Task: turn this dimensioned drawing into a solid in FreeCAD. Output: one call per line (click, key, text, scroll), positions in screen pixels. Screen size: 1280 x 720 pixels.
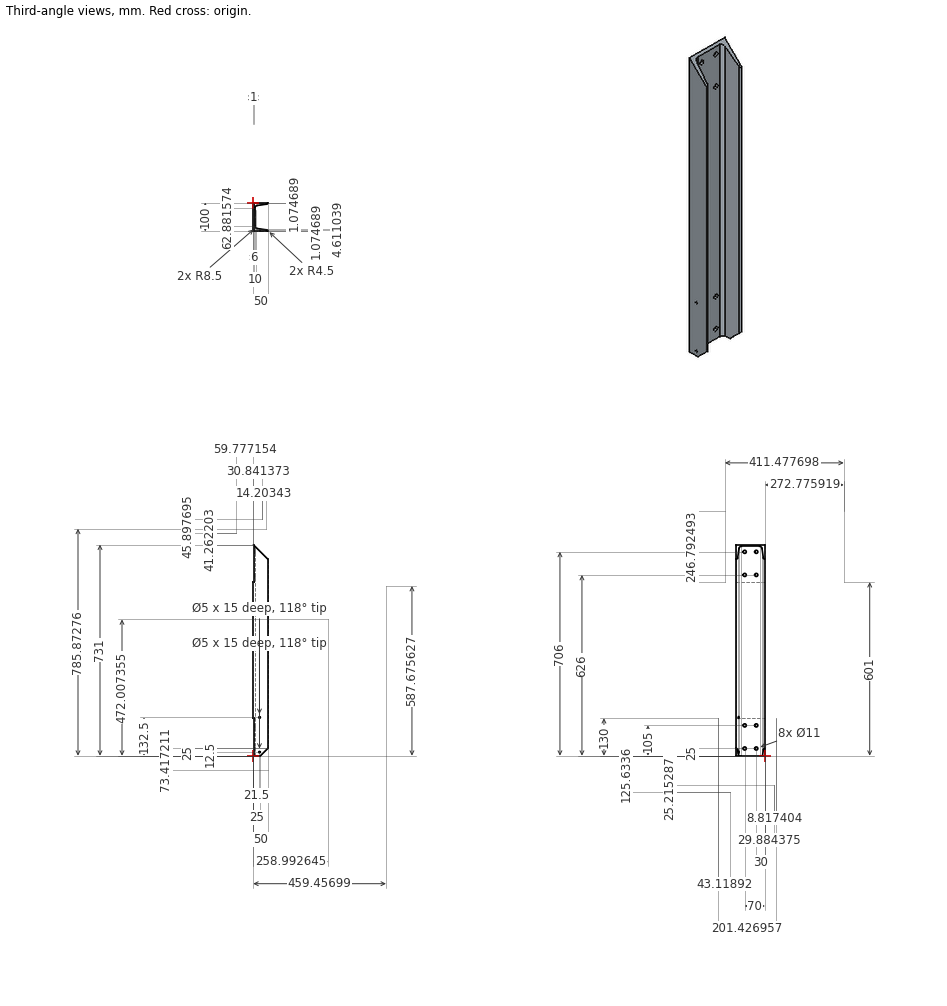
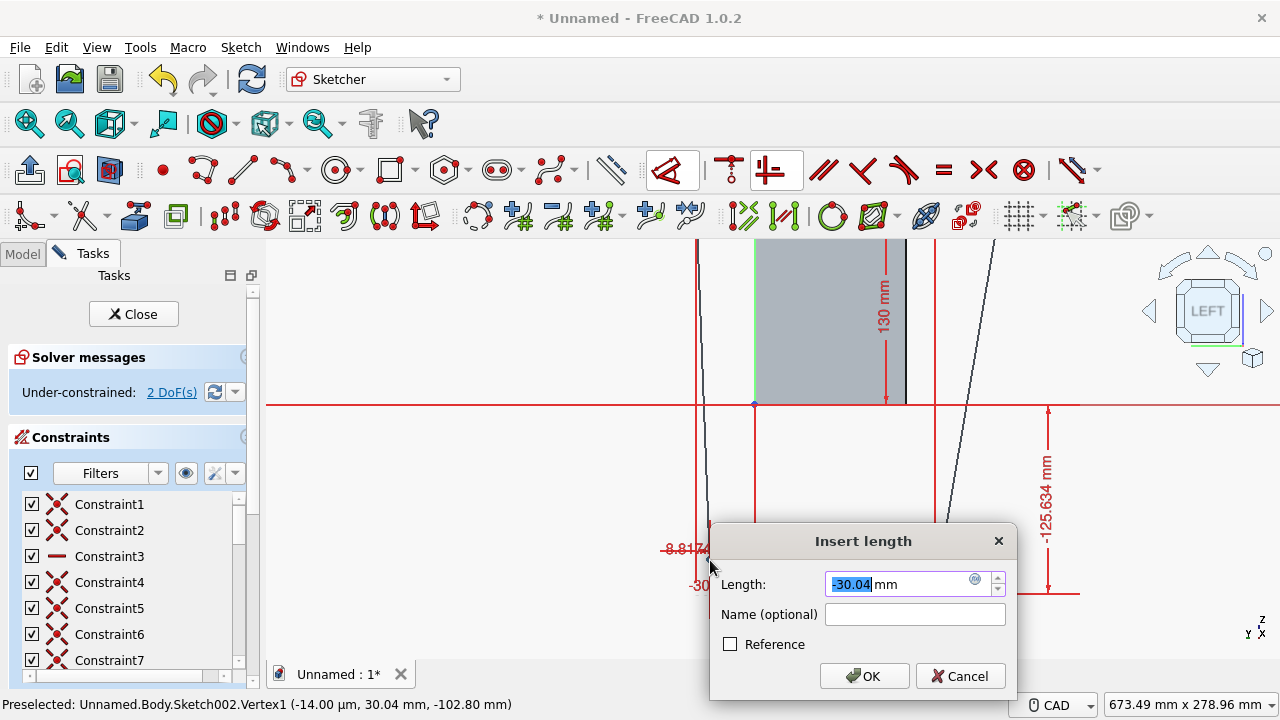
text(-29.884375)
key(Return)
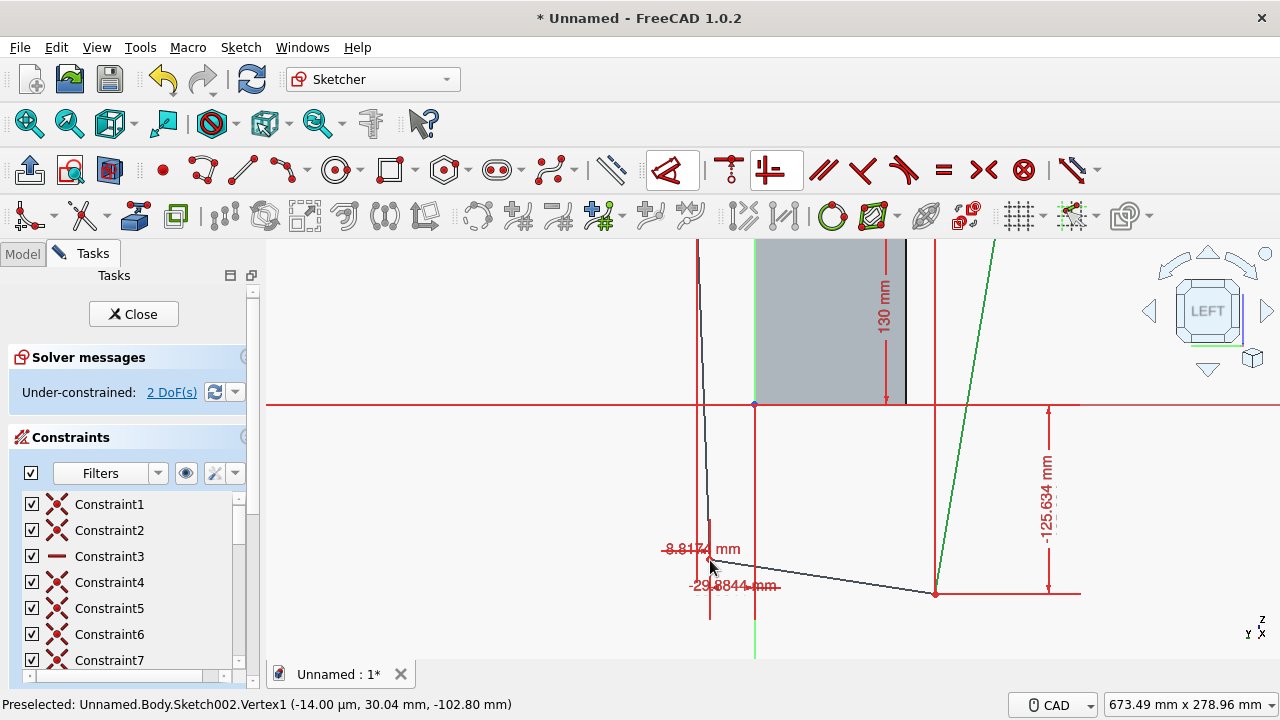
click(777, 570)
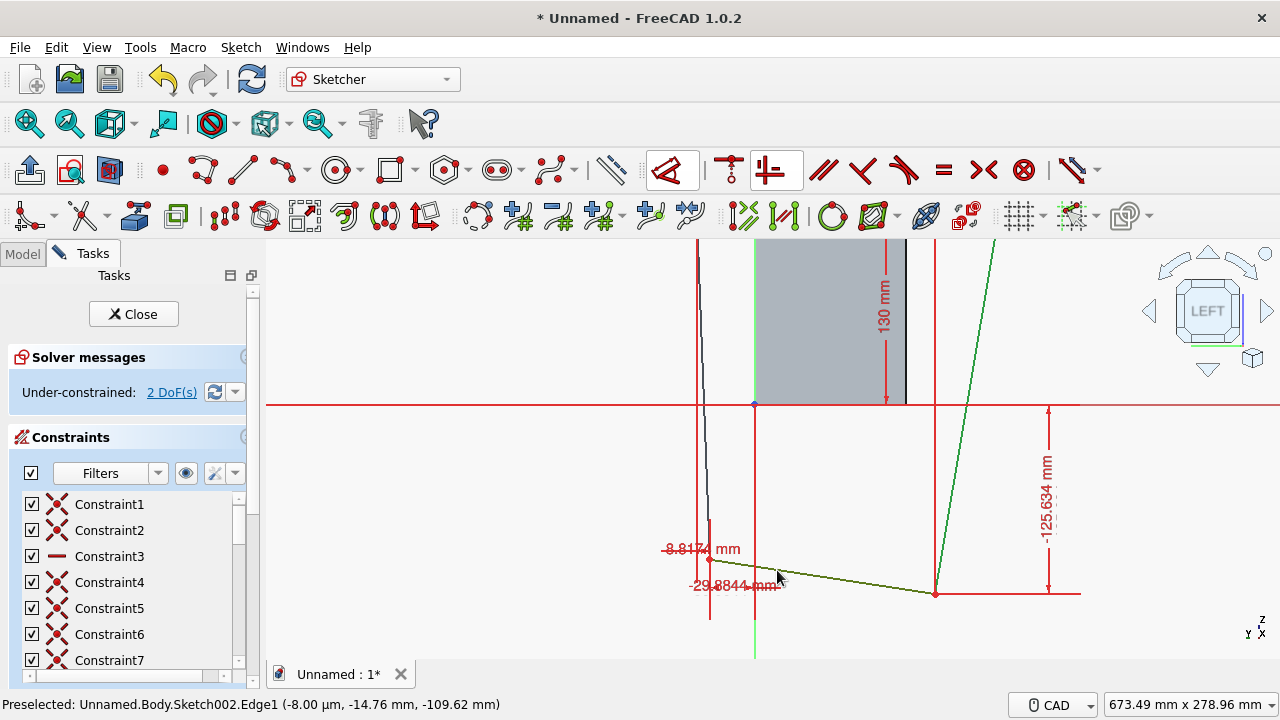
click(694, 170)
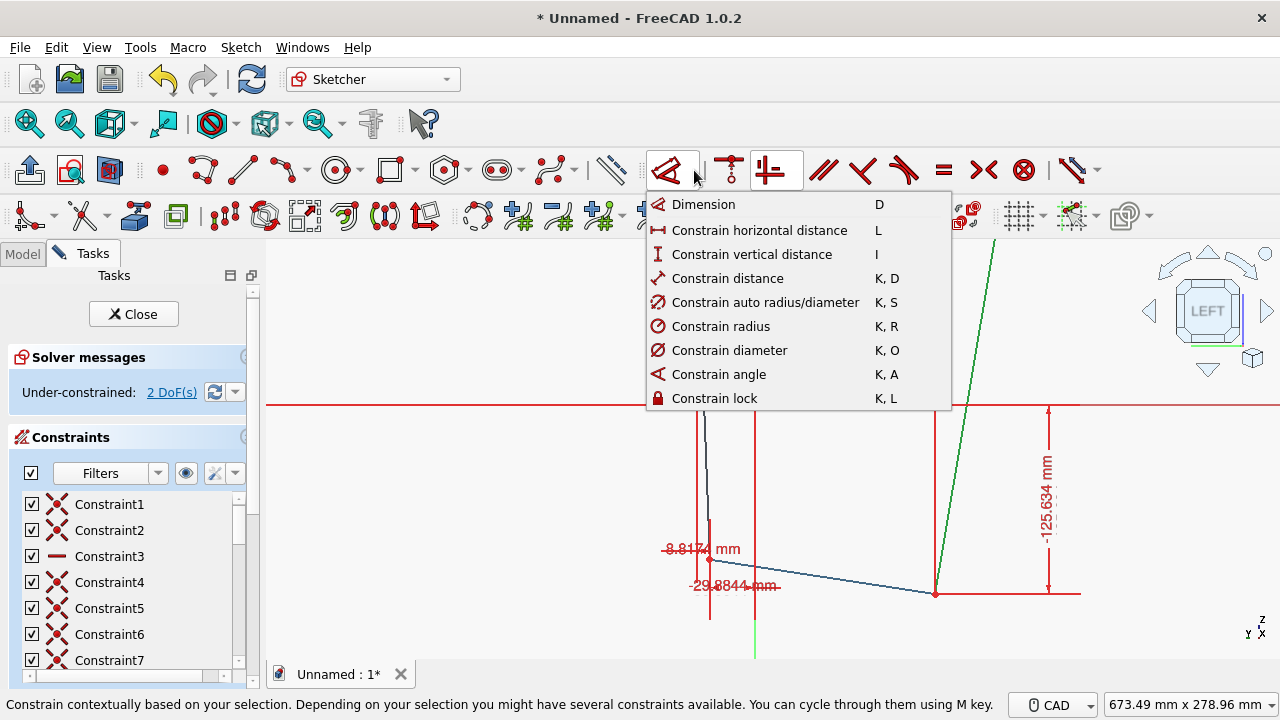
click(799, 254)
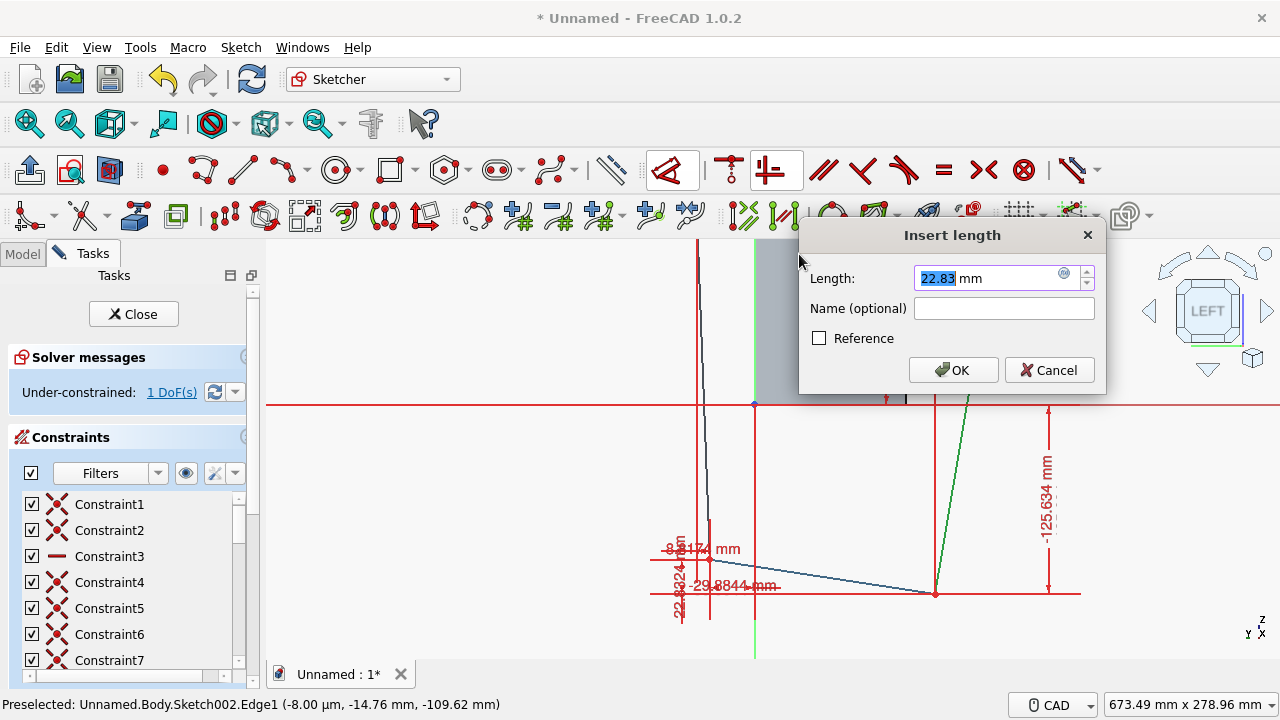
text(25.215287)
key(Return)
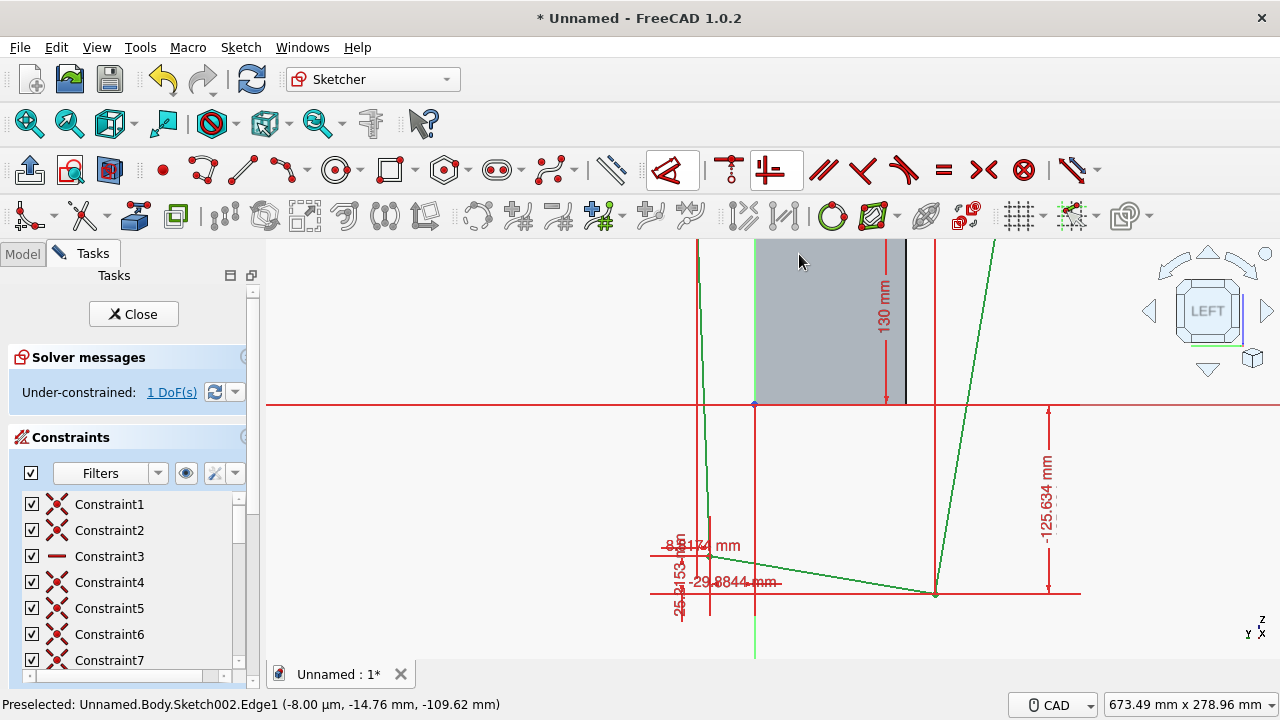
scroll(711, 565, down, 9)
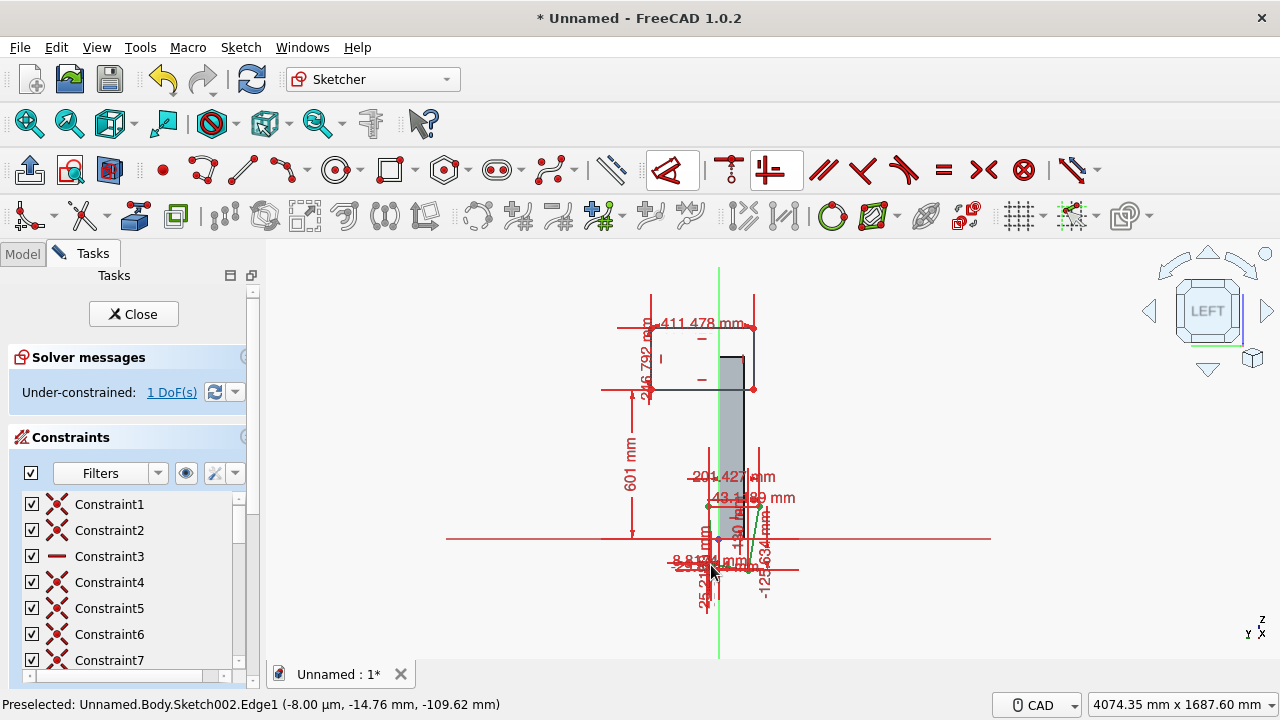
click(651, 328)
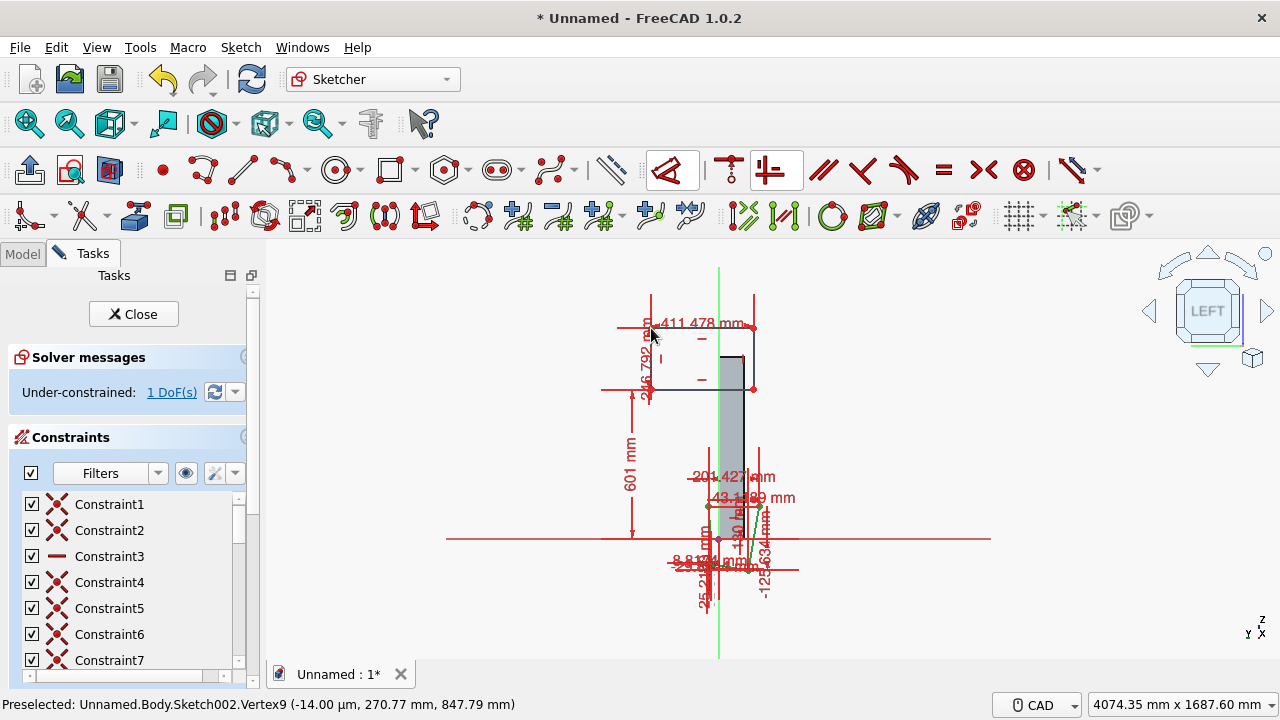
key(l)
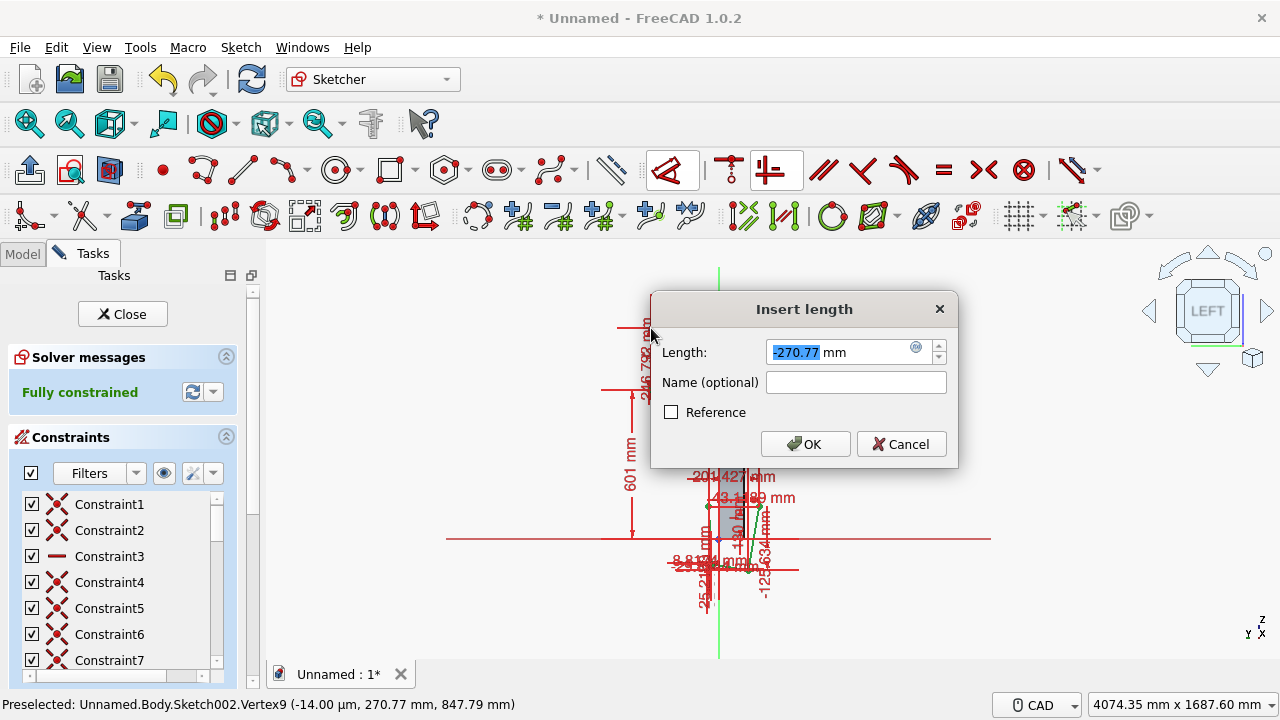
text(-272.775919)
key(Return)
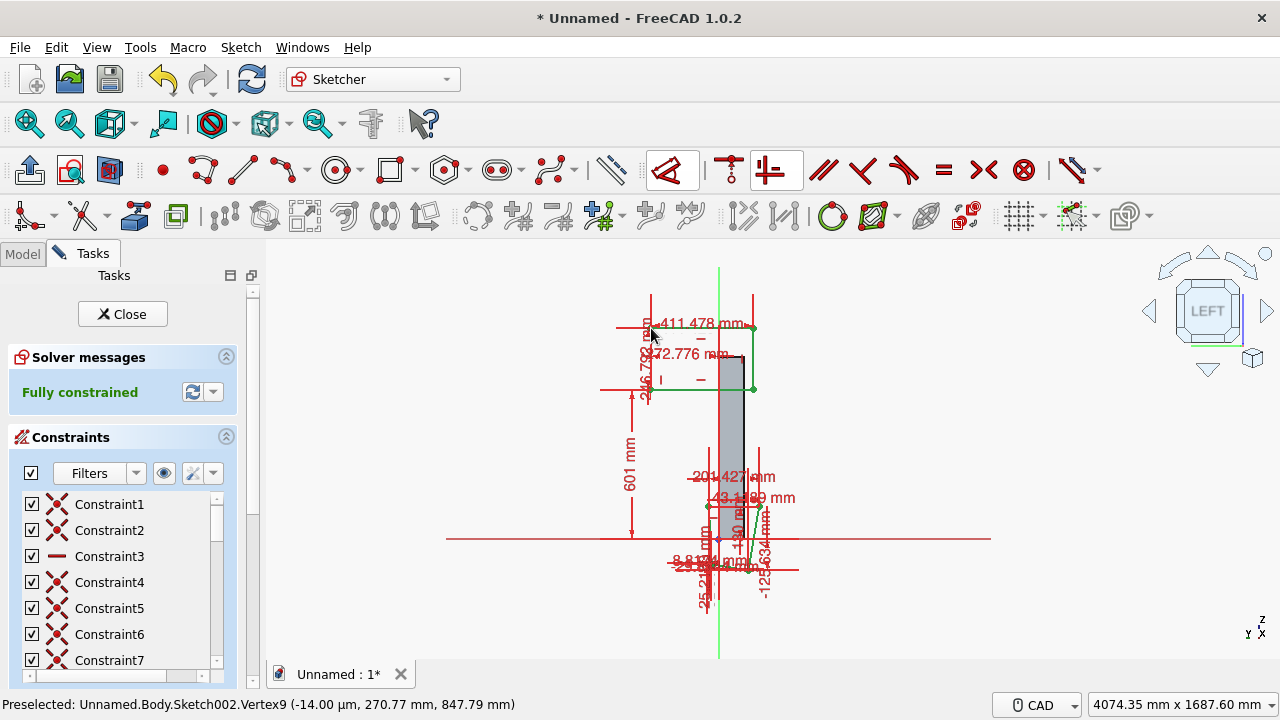
click(123, 314)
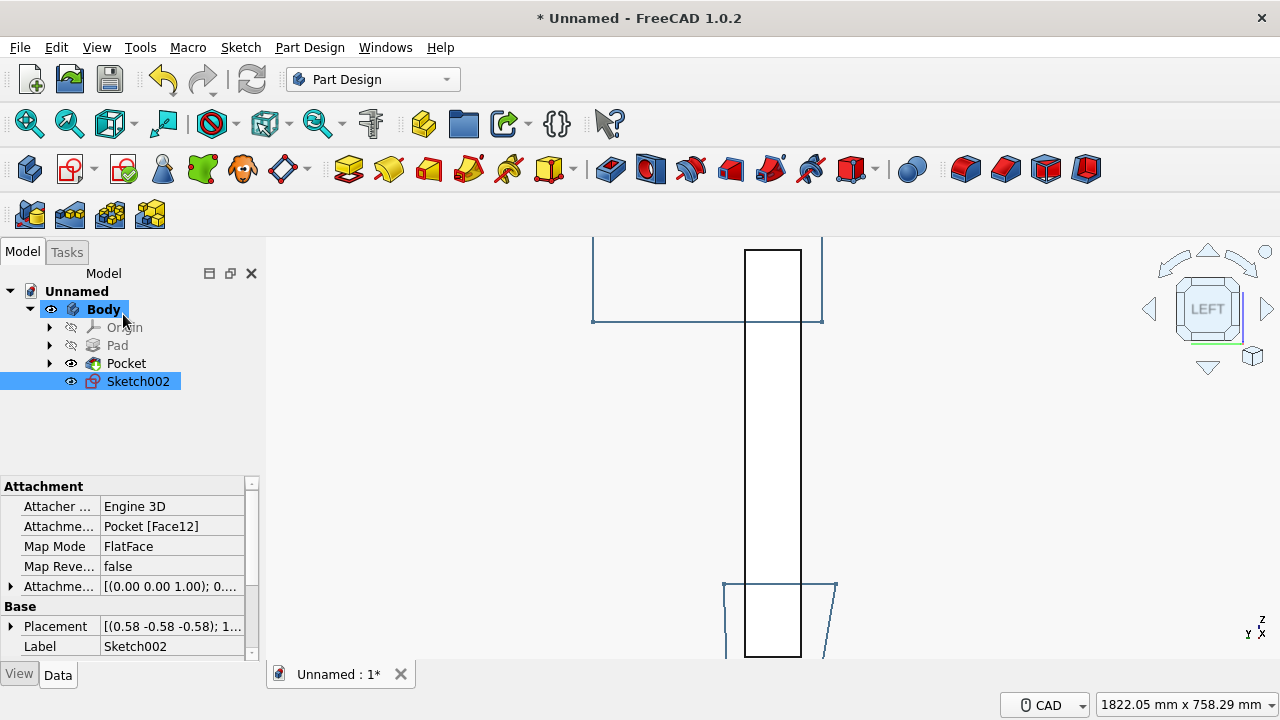
click(612, 170)